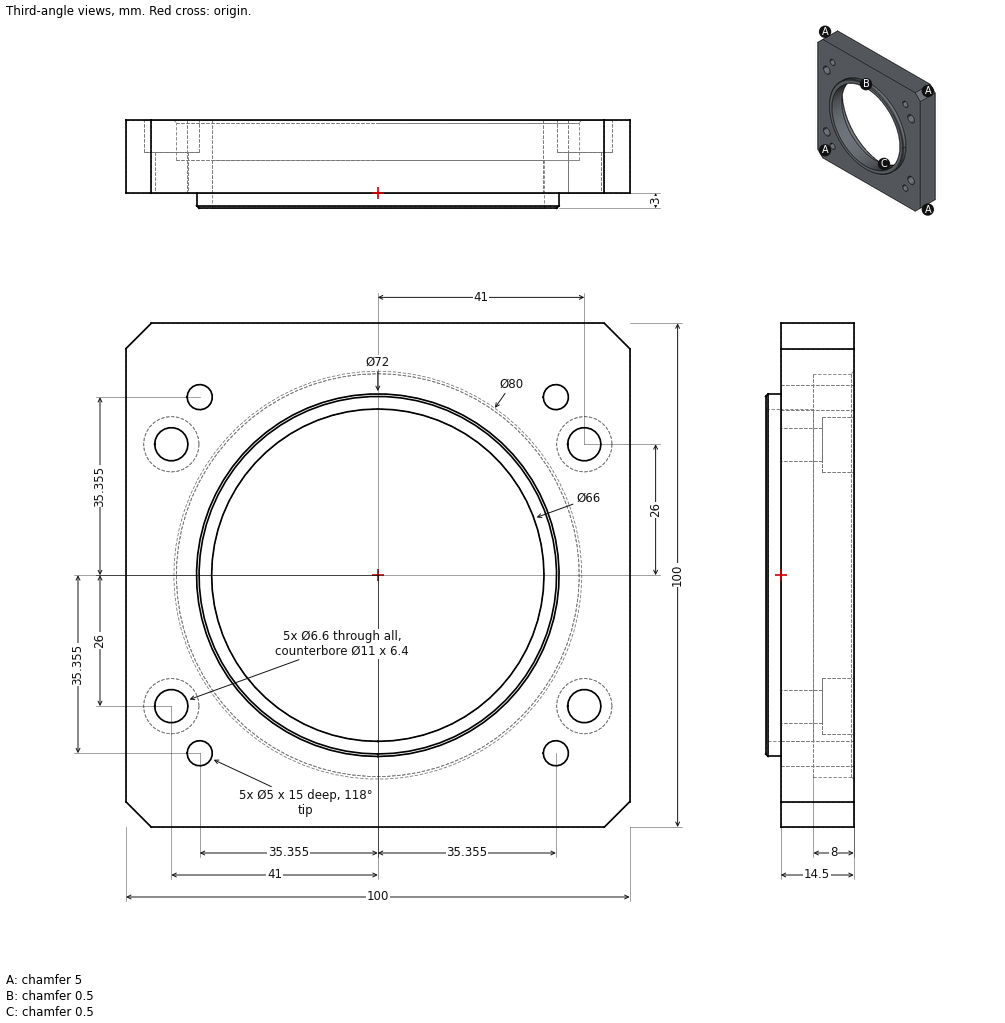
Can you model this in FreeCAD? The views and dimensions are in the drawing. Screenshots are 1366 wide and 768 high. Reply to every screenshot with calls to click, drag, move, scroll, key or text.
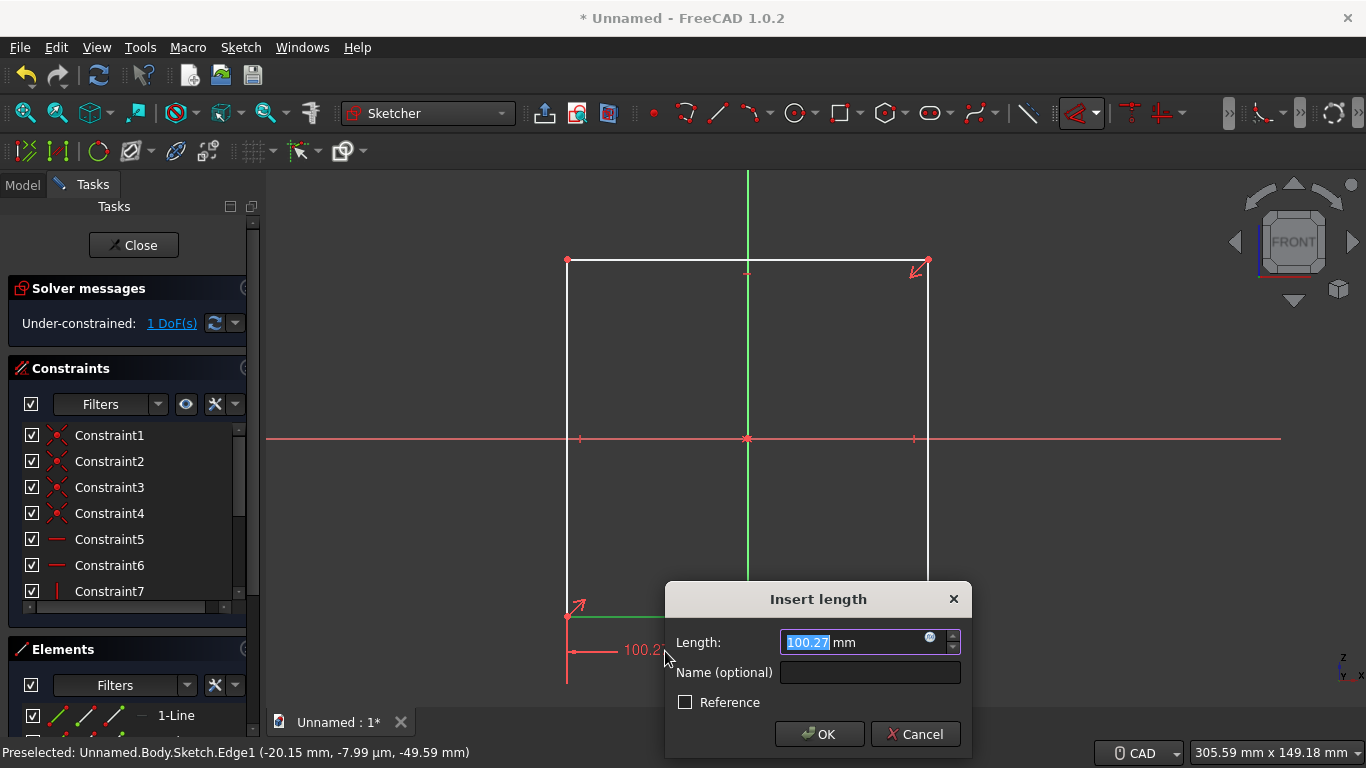
text(100)
key(Return)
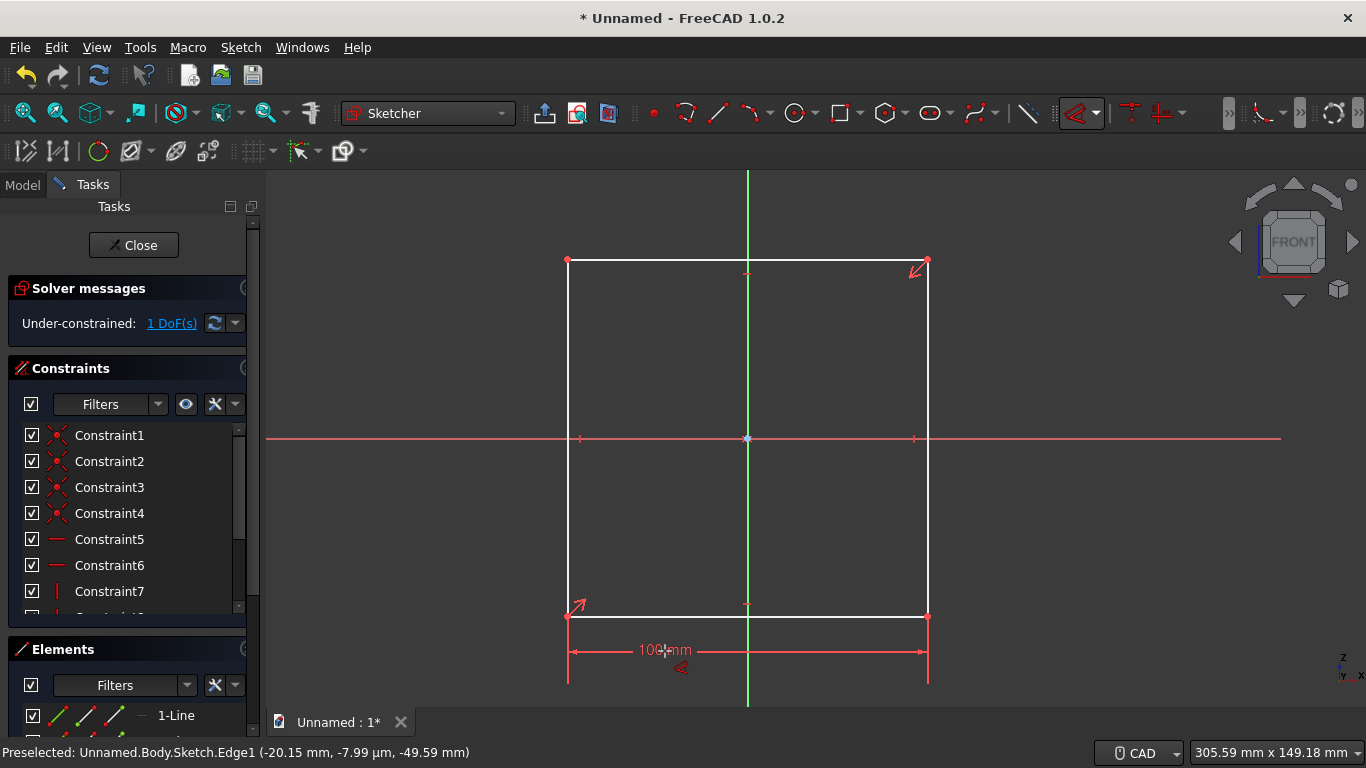
click(928, 510)
click(962, 356)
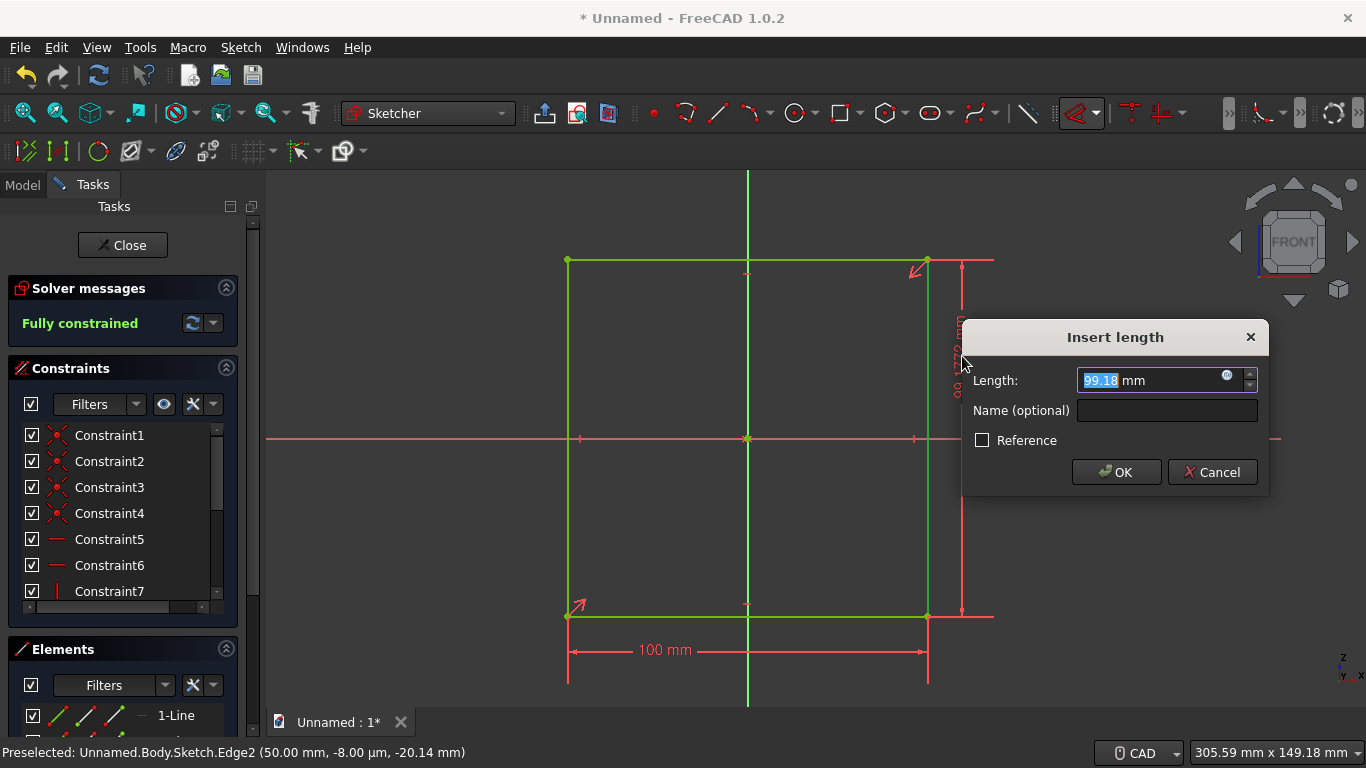
text(100)
key(Return)
key(Escape)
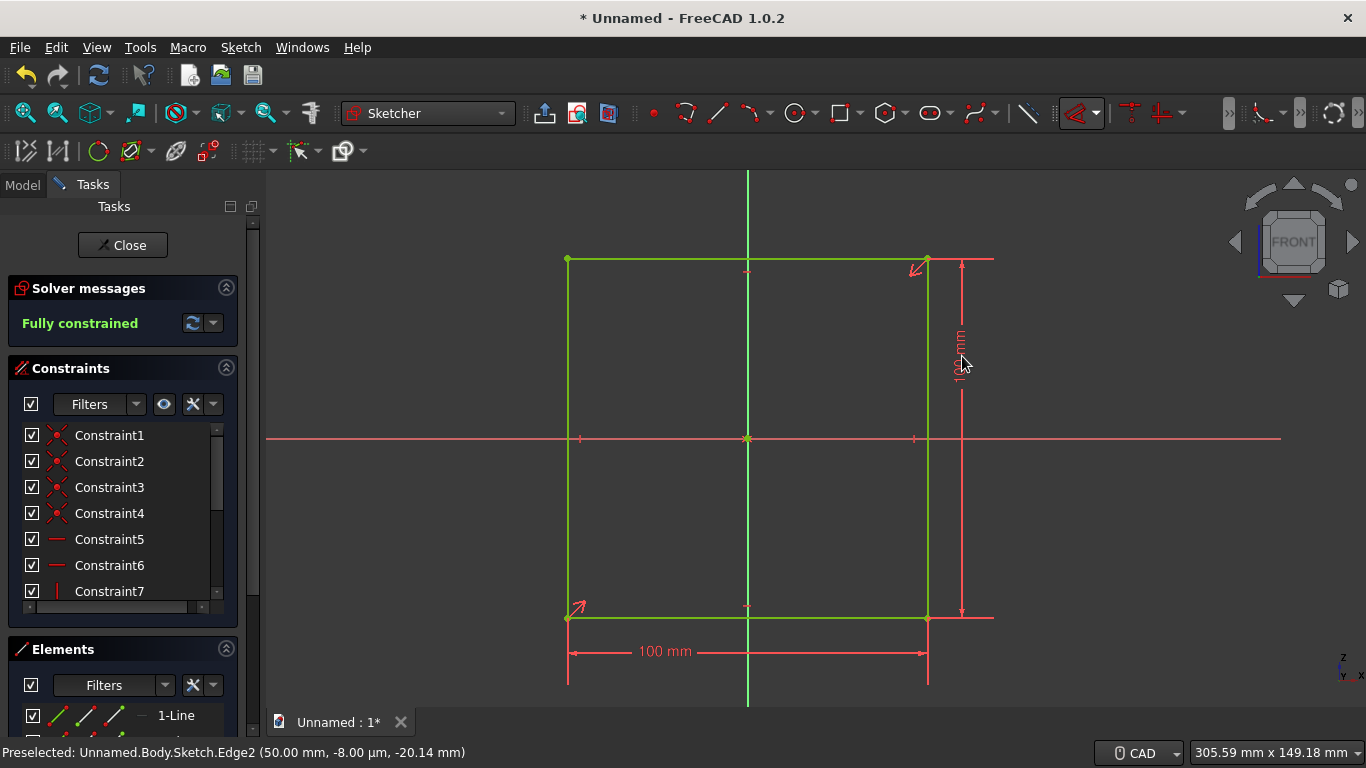
click(123, 245)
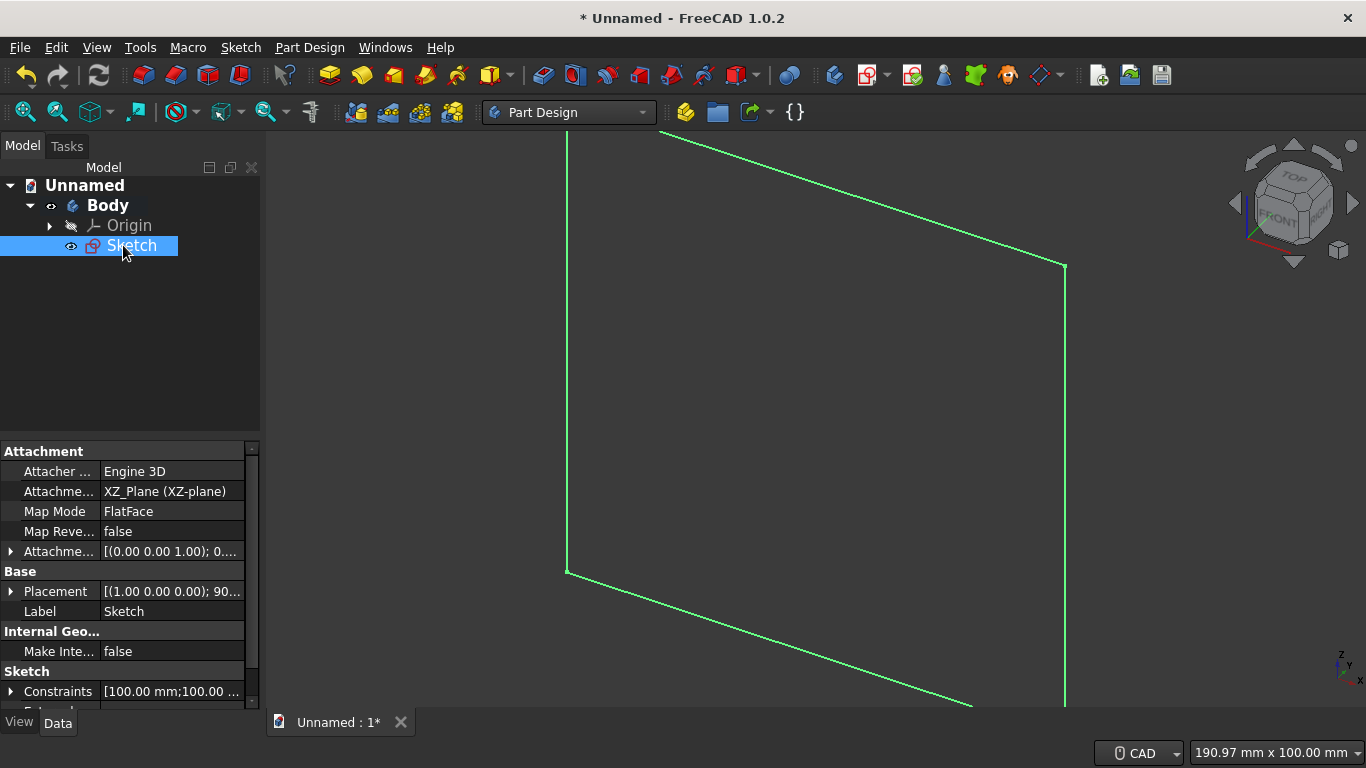
click(330, 76)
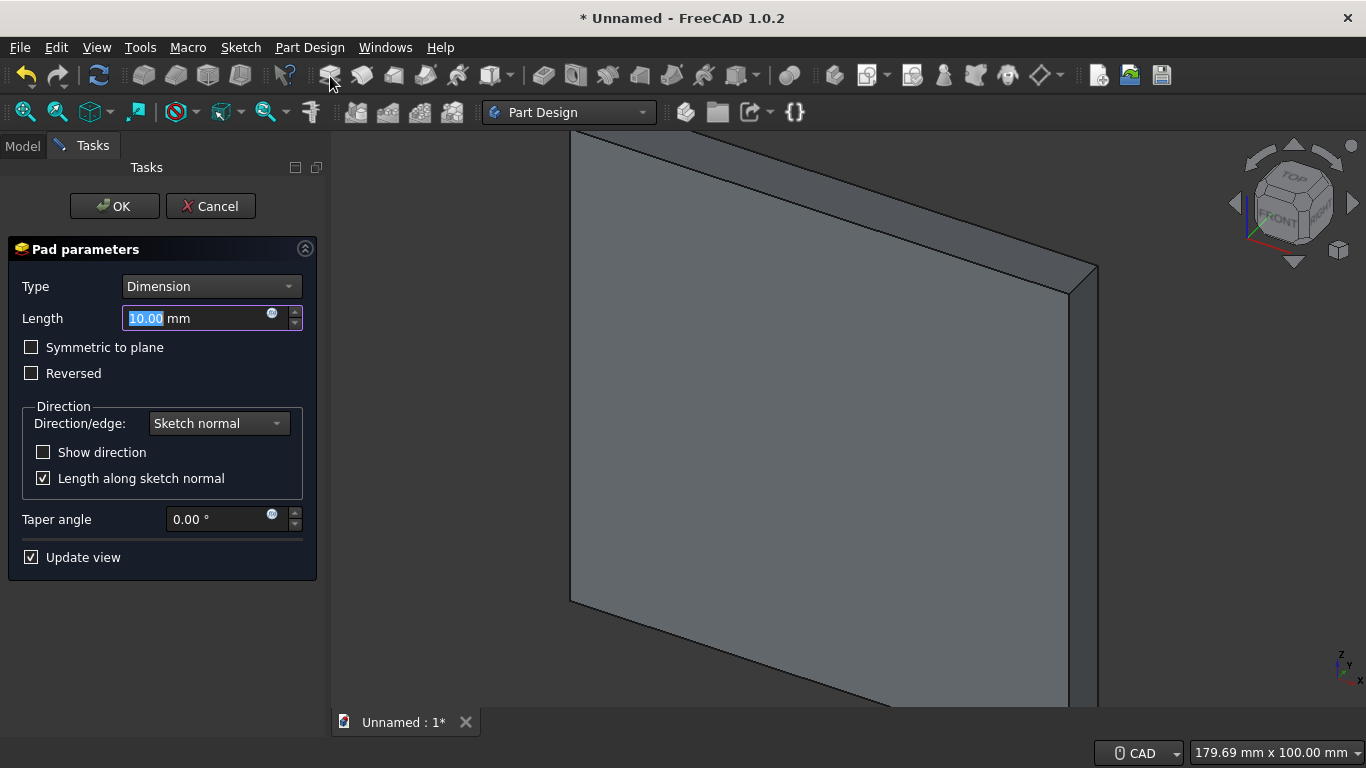
text(14.5)
key(Tab)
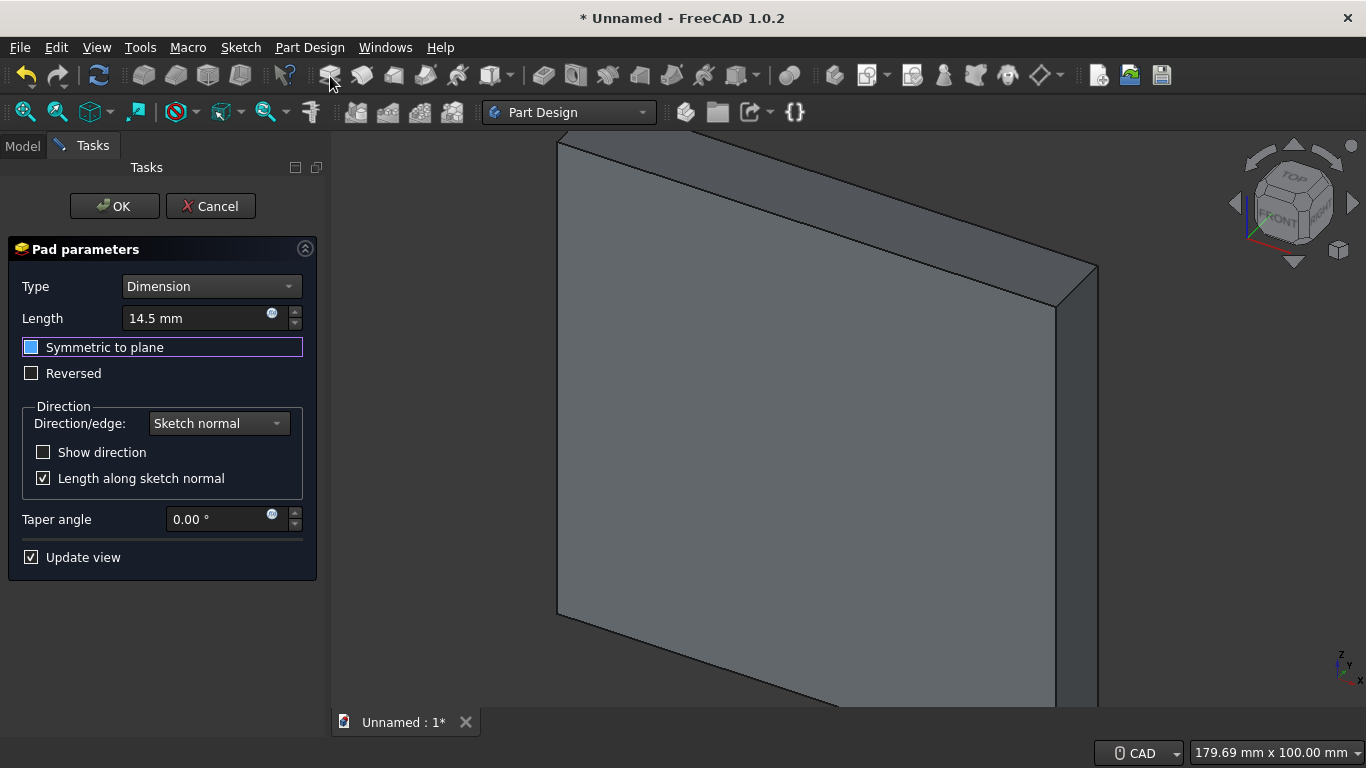
click(30, 373)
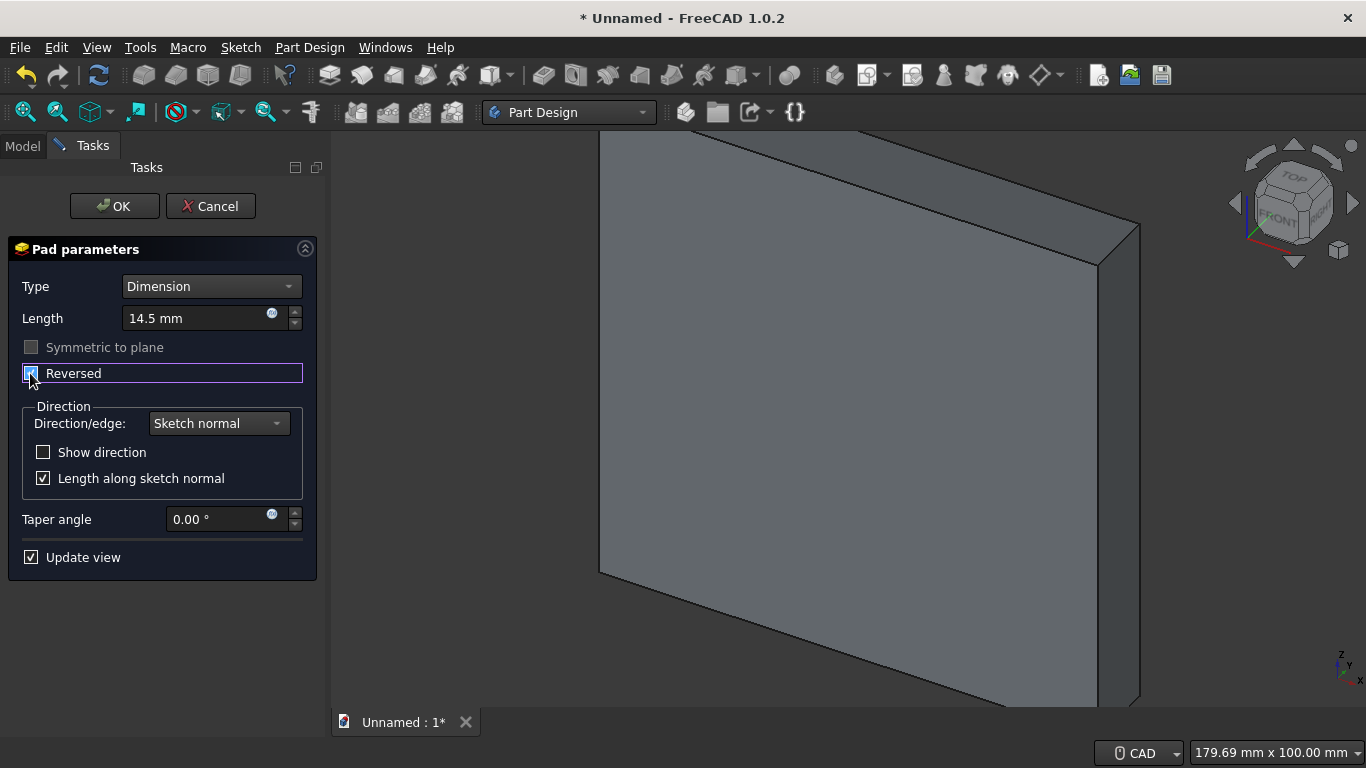
click(115, 206)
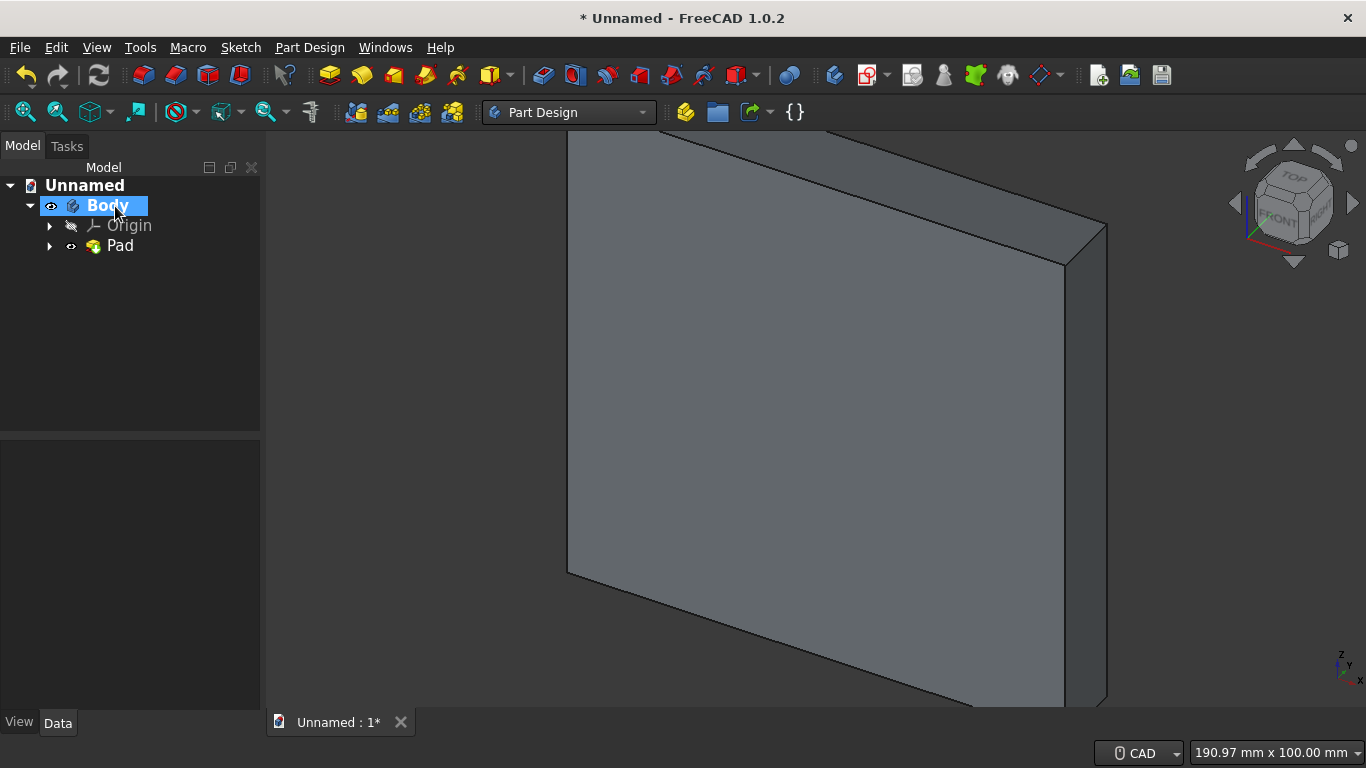
key(v)
key(f)